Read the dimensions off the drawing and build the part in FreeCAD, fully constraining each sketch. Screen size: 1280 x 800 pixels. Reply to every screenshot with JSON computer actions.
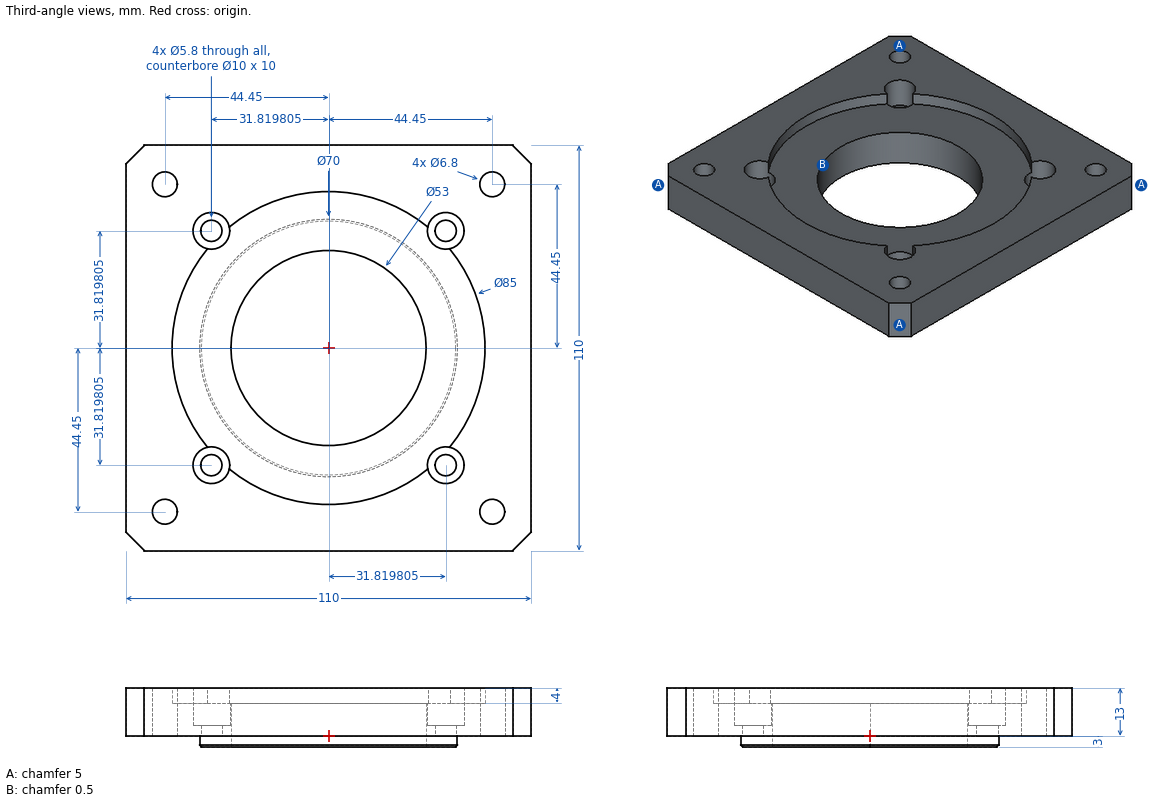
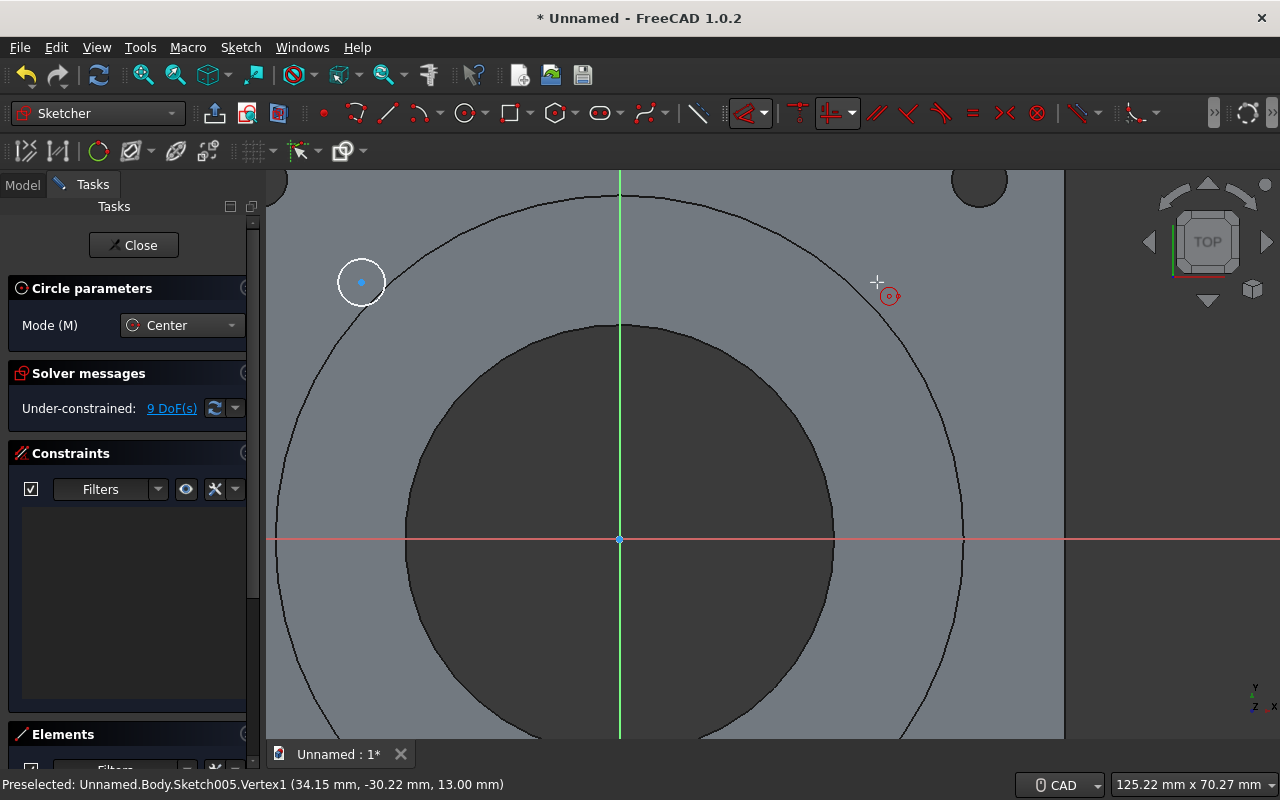
{"action": "left_click", "coordinate": [877, 282]}
{"action": "left_click", "coordinate": [894, 265]}
{"action": "key", "text": "Escape"}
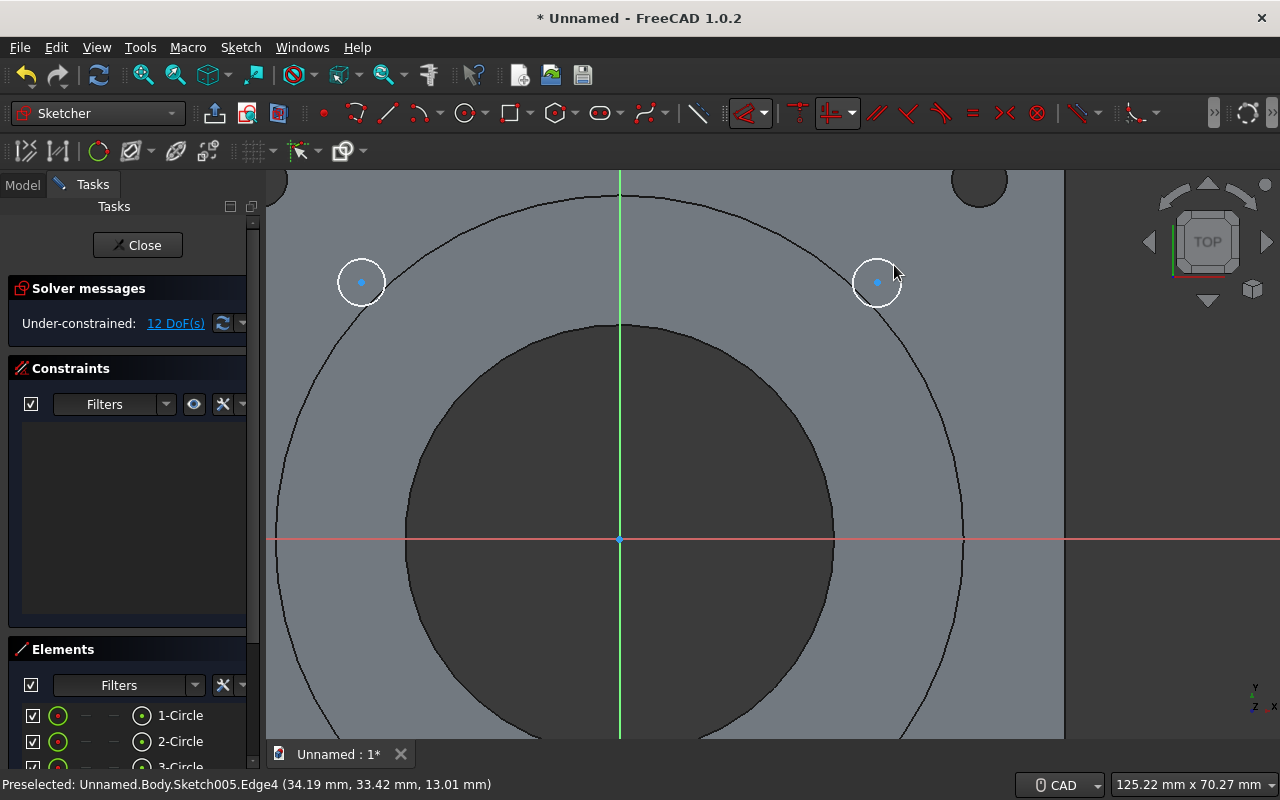
{"action": "left_click", "coordinate": [378, 266]}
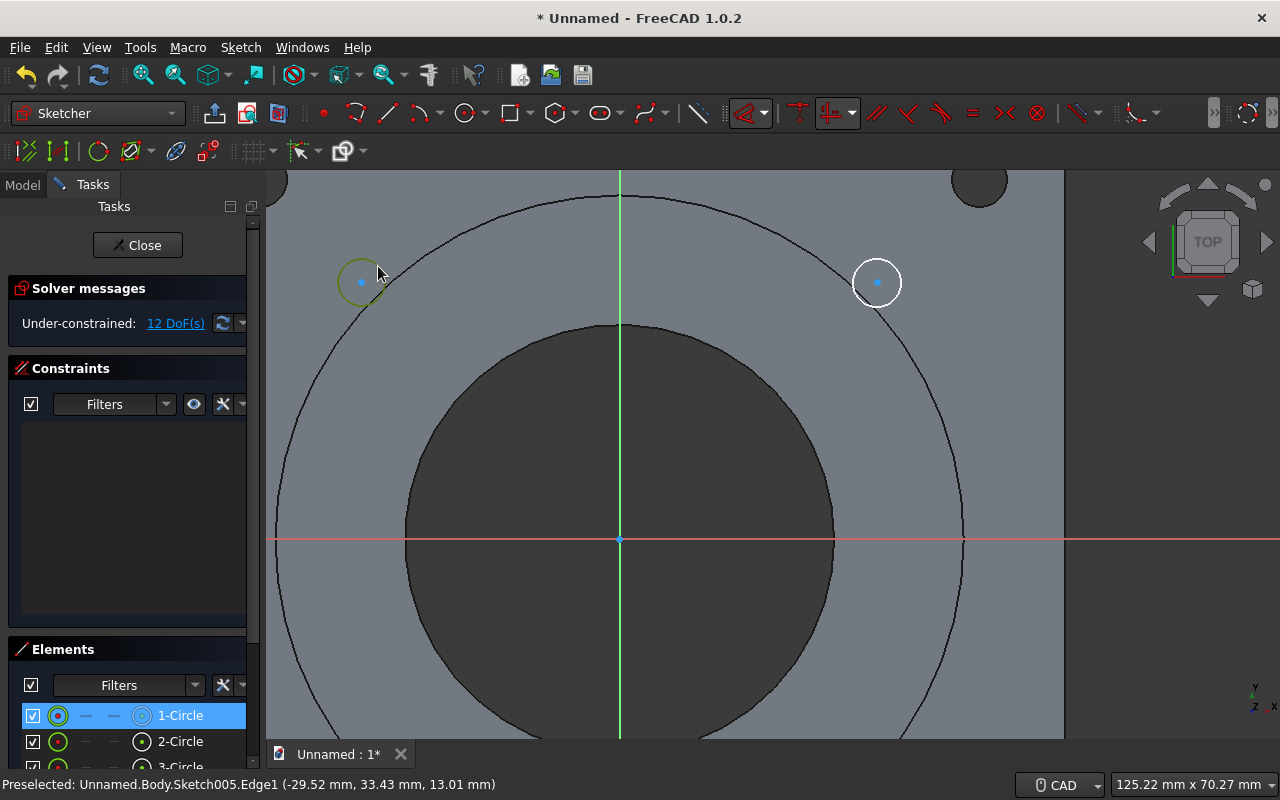
{"action": "scroll", "coordinate": [877, 282], "scroll_direction": "down", "scroll_amount": 2}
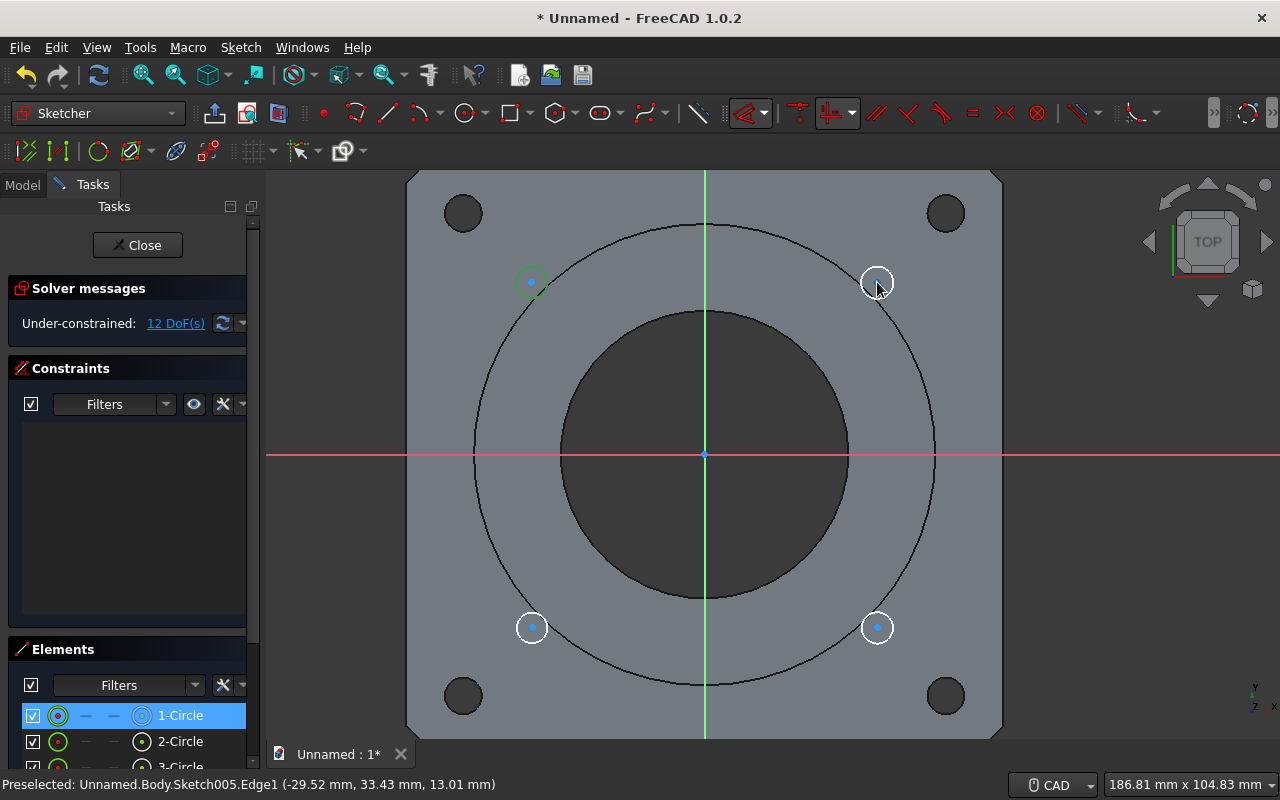
{"action": "left_click", "coordinate": [543, 617]}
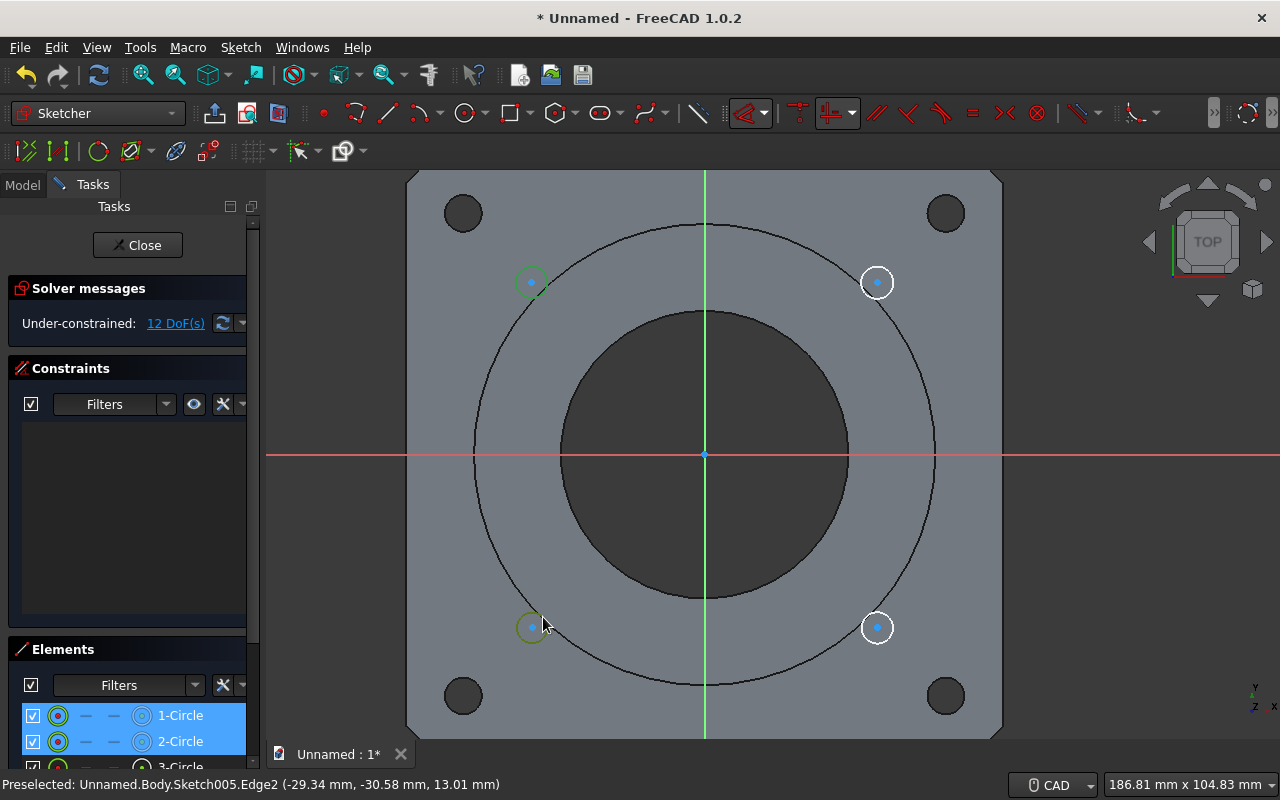
{"action": "left_click", "coordinate": [888, 617]}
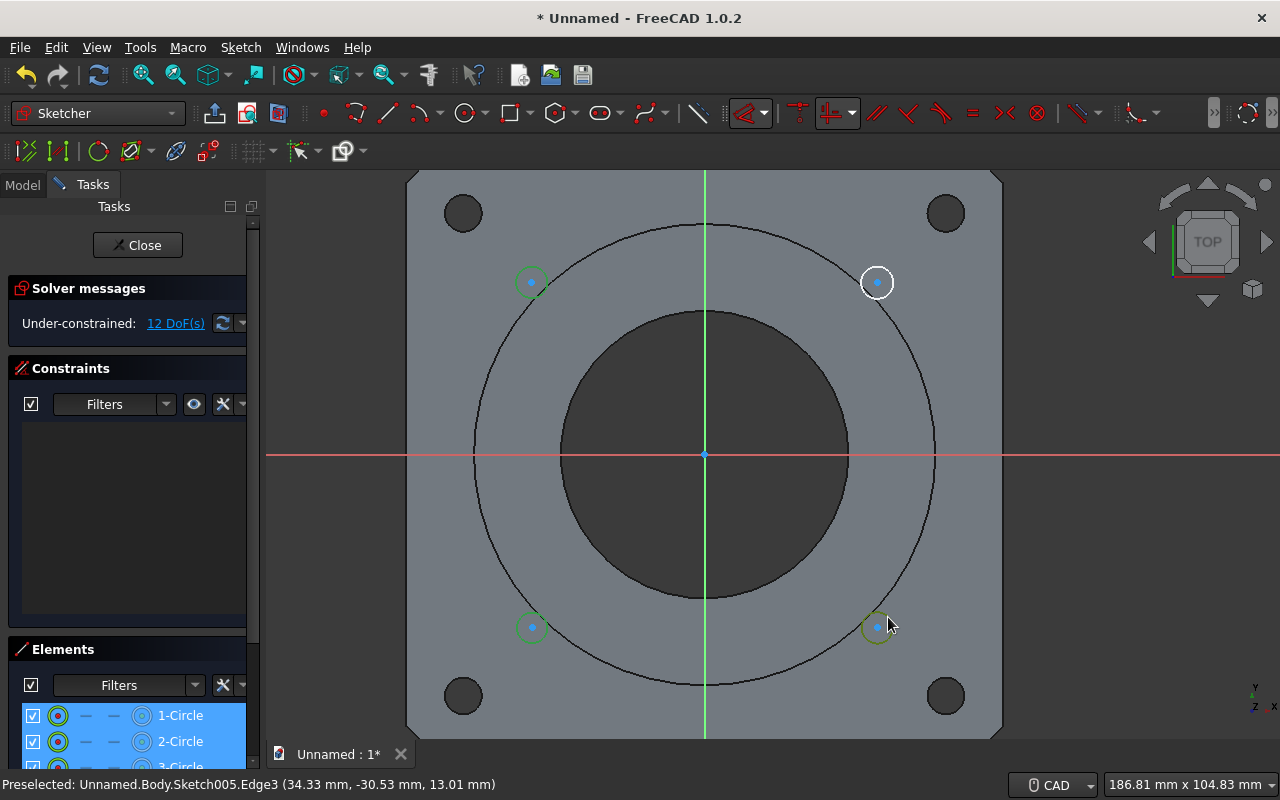
{"action": "left_click", "coordinate": [889, 271]}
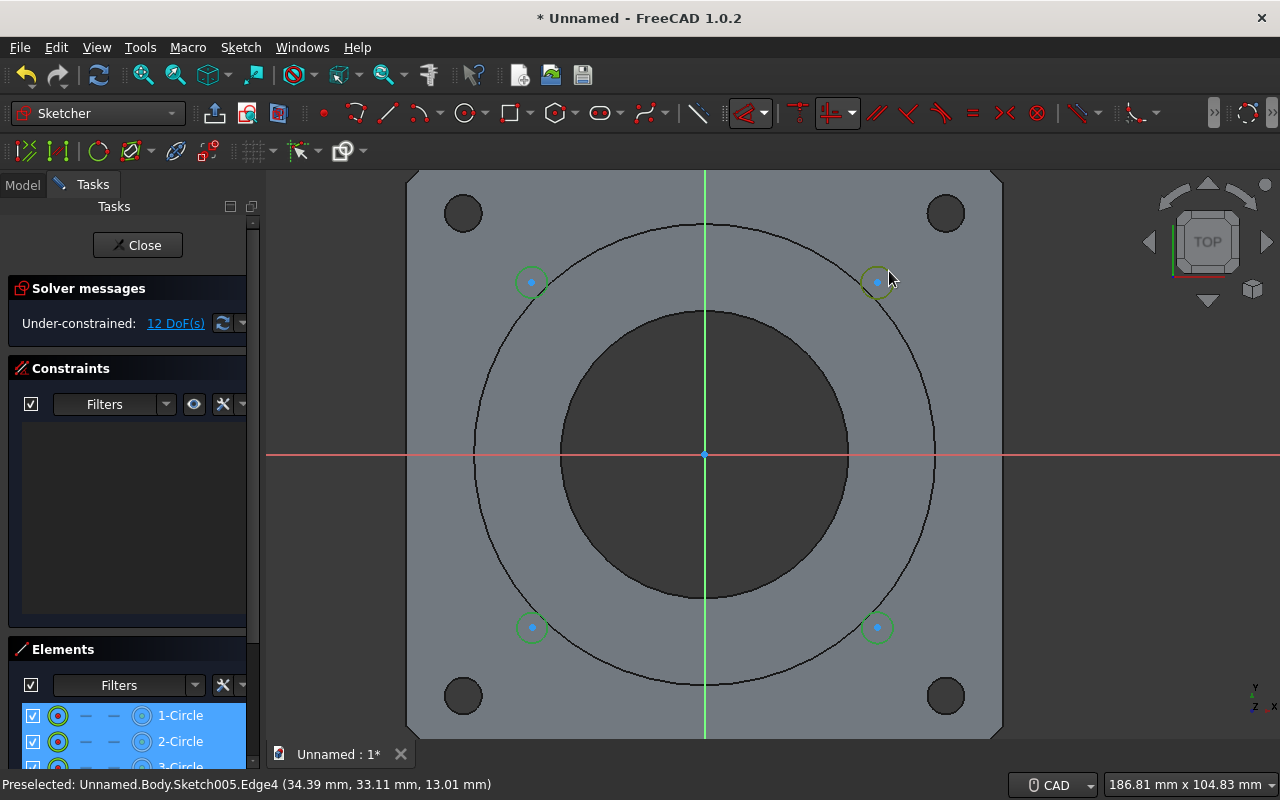
{"action": "left_click", "coordinate": [974, 114]}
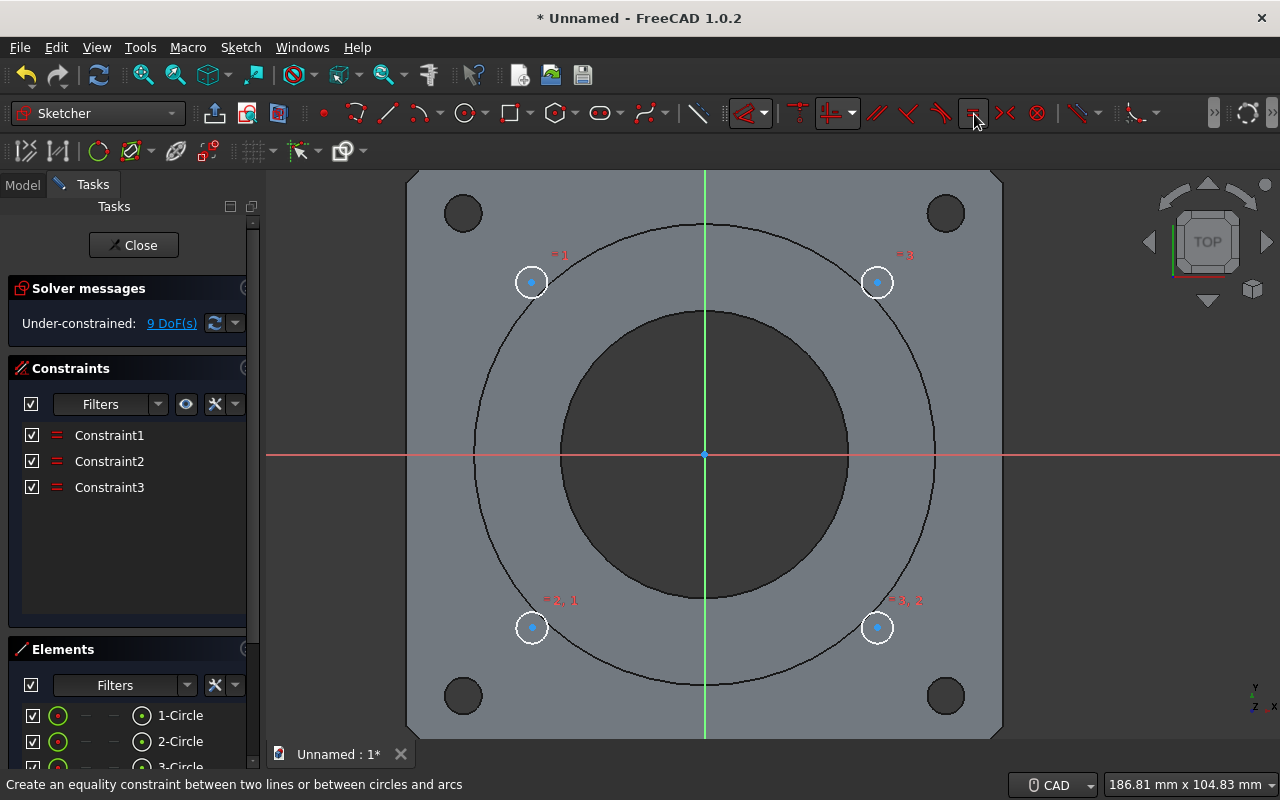
{"action": "left_click", "coordinate": [532, 282]}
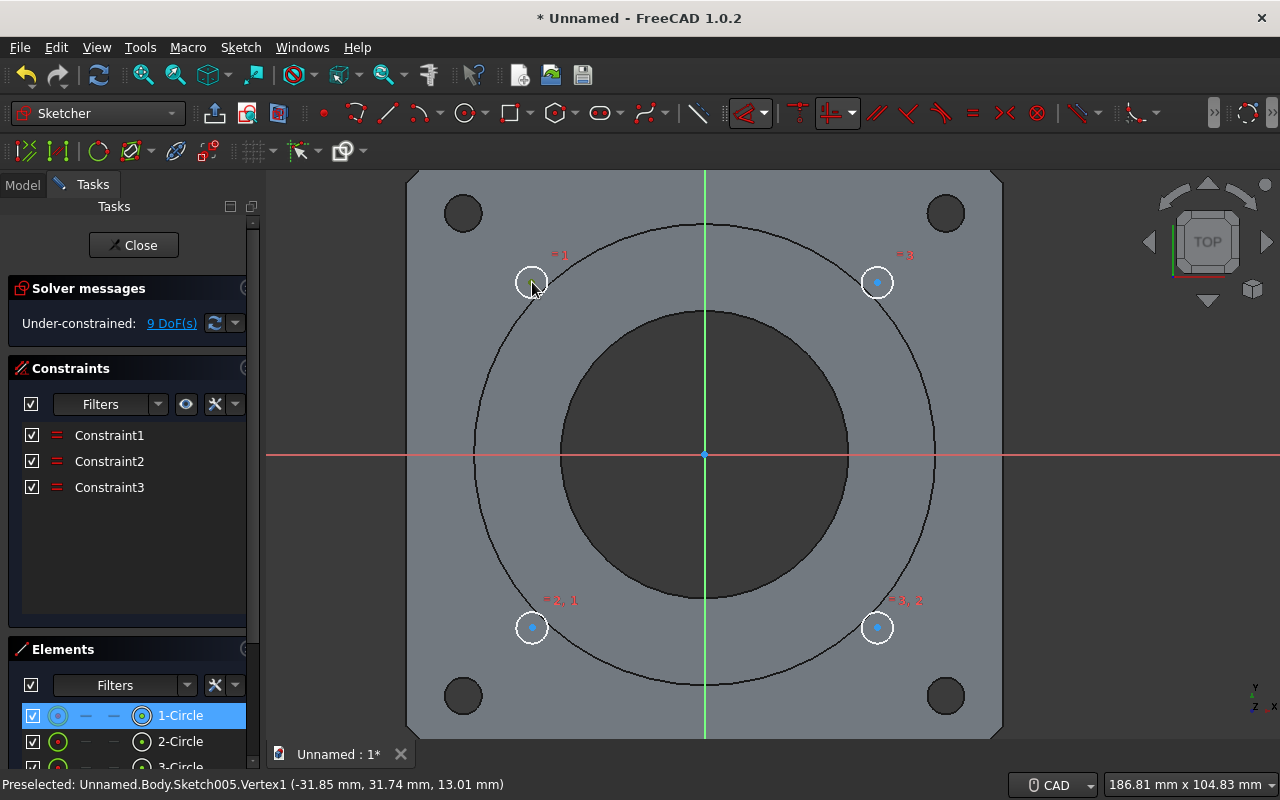
{"action": "left_click", "coordinate": [532, 628]}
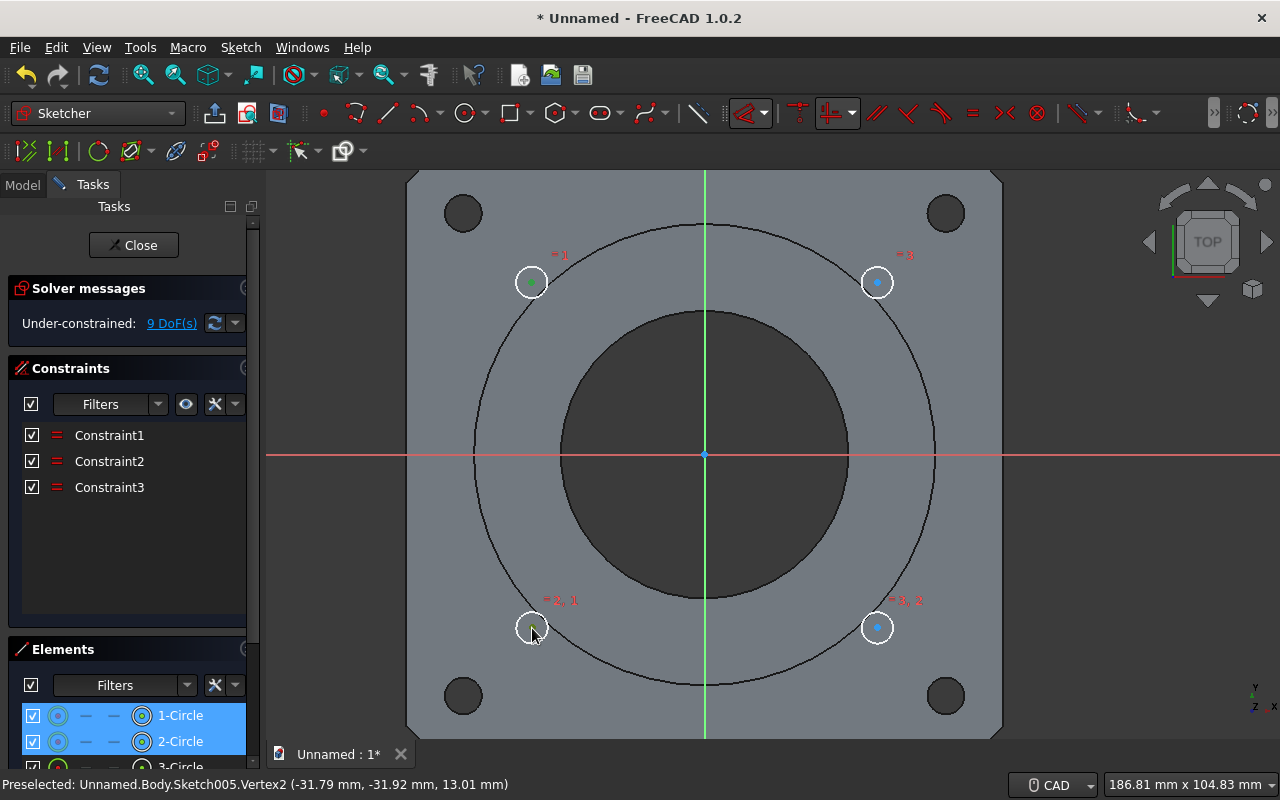
{"action": "left_click", "coordinate": [854, 114]}